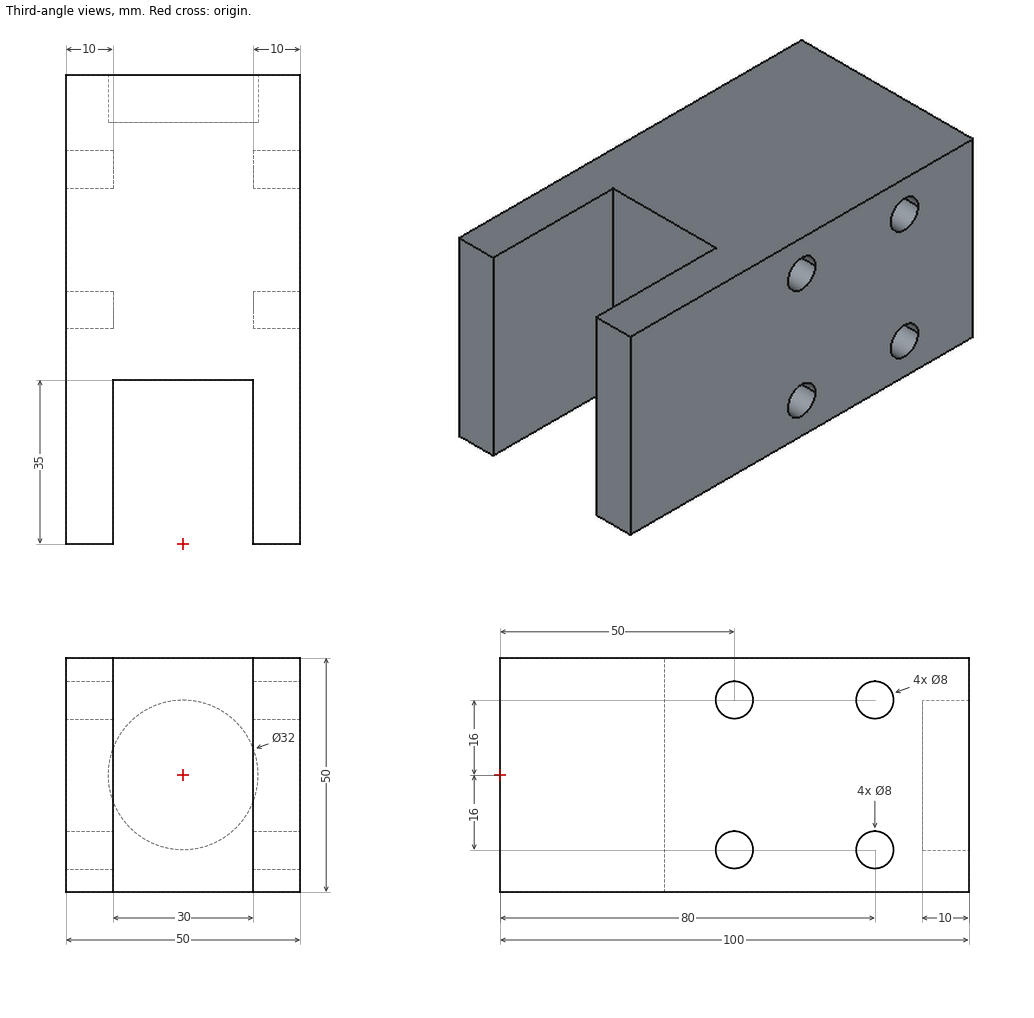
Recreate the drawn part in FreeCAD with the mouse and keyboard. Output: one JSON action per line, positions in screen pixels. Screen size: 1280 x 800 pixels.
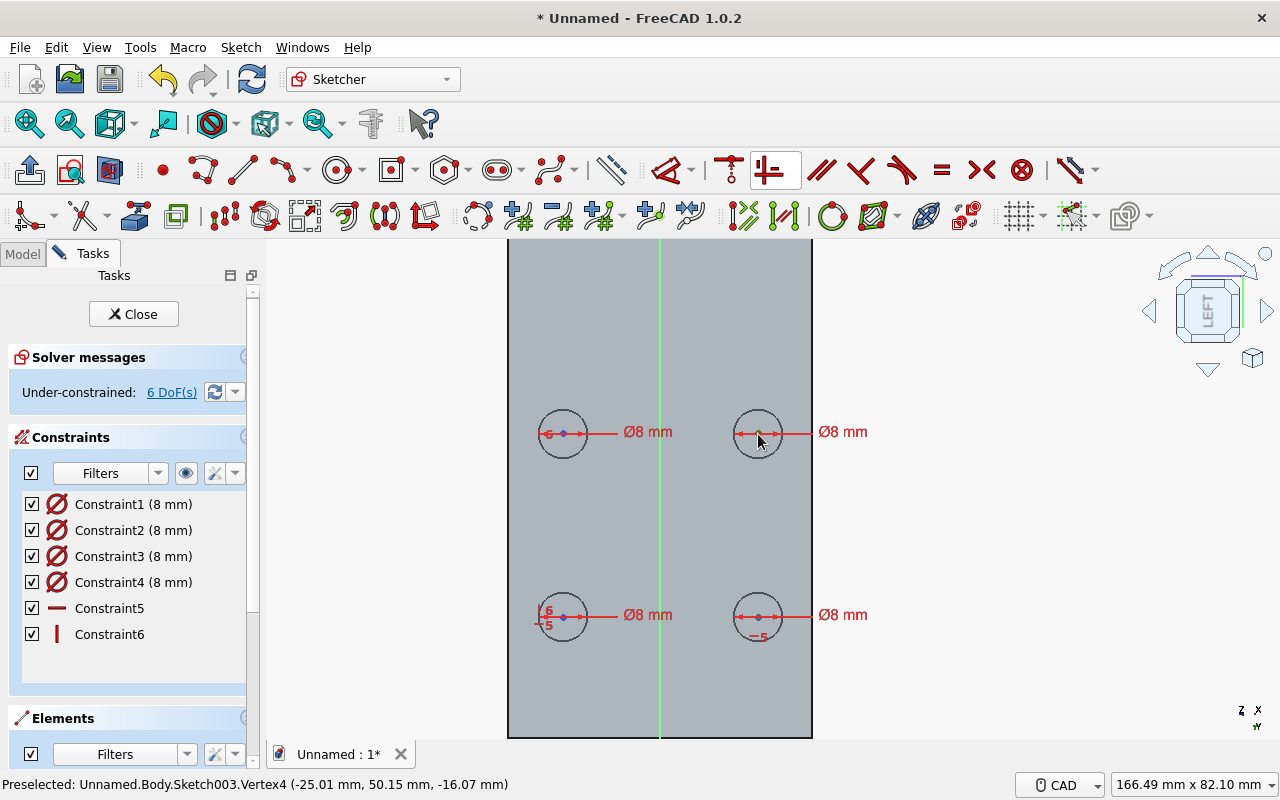
{"action": "left_click", "coordinate": [796, 170]}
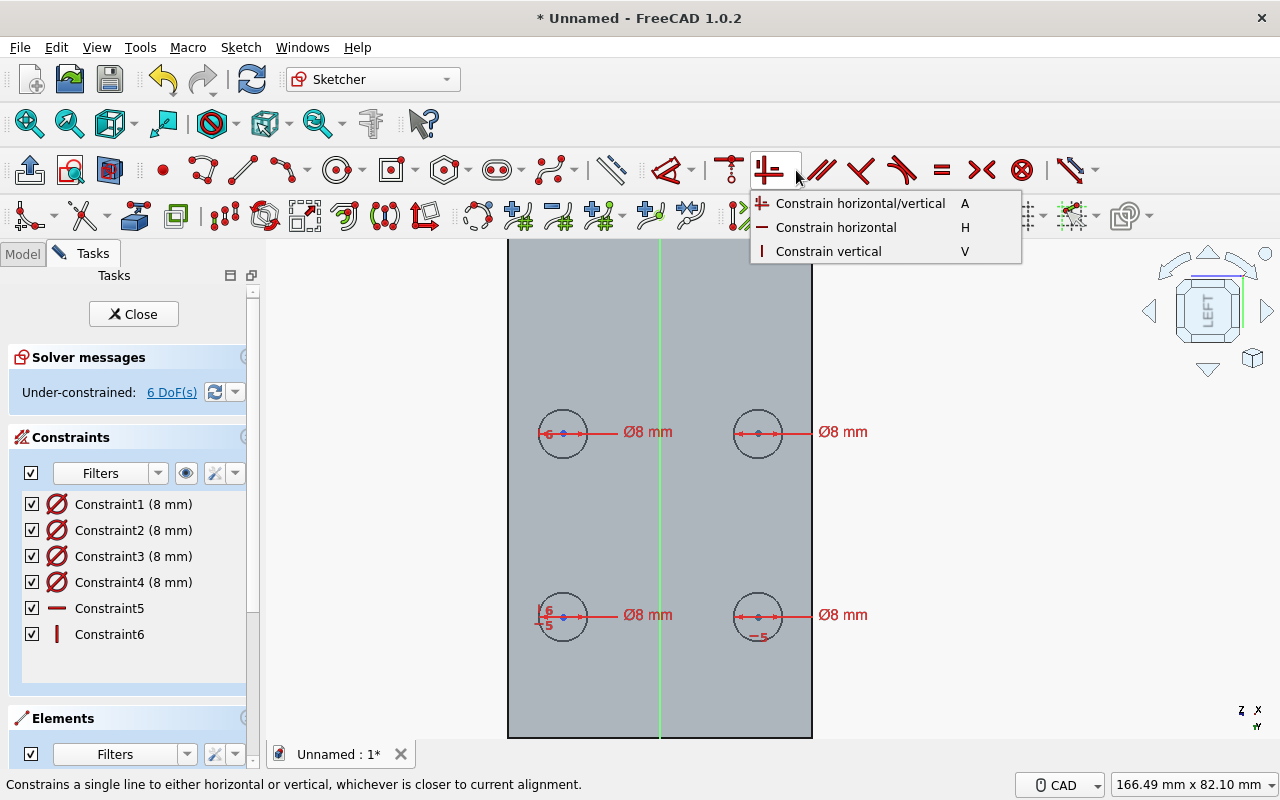
{"action": "left_click", "coordinate": [886, 251]}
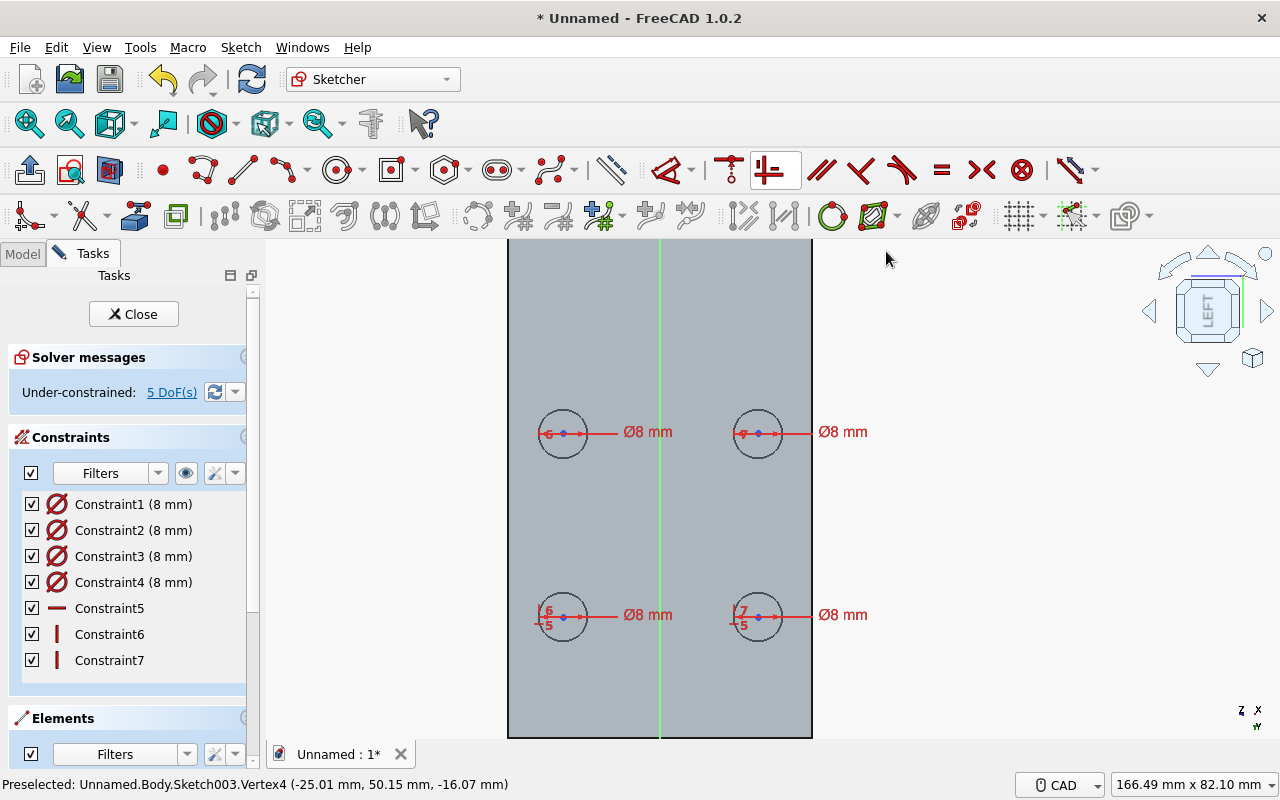
{"action": "left_click", "coordinate": [563, 434]}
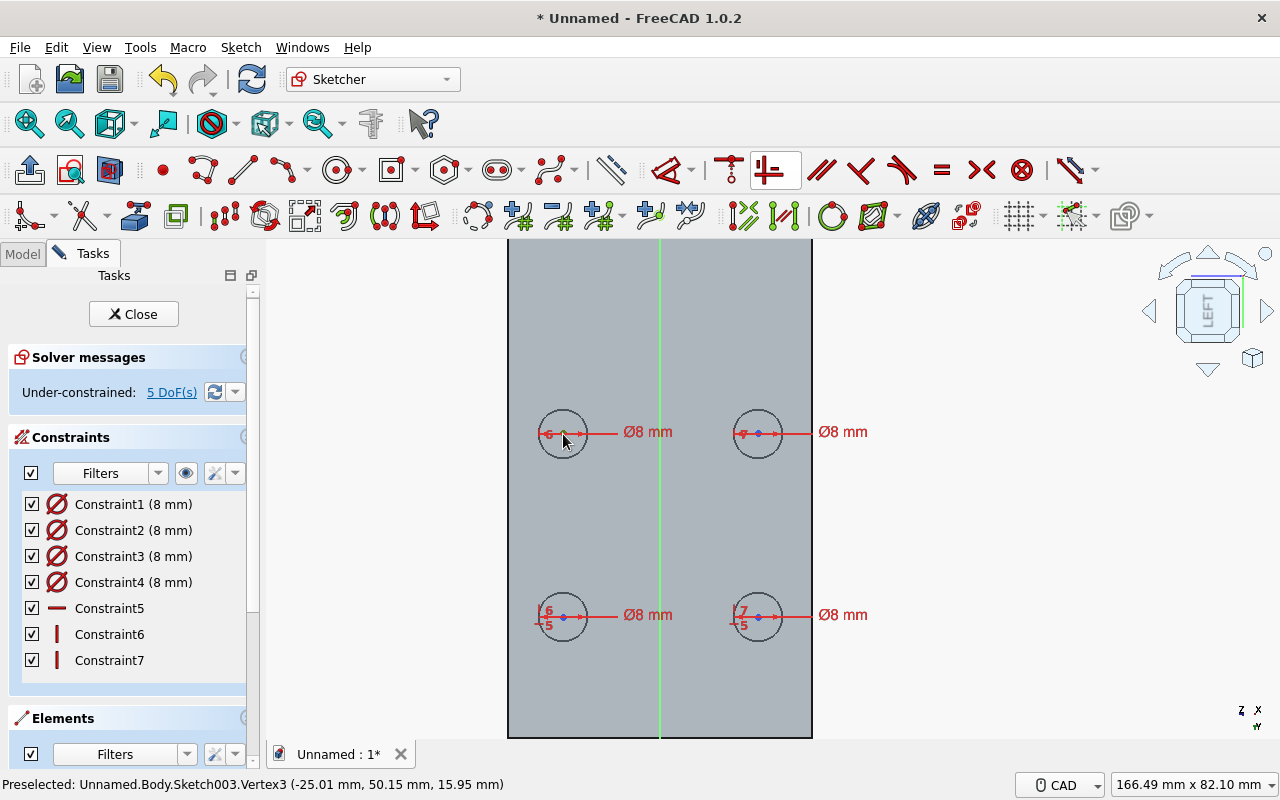
{"action": "left_click", "coordinate": [758, 434]}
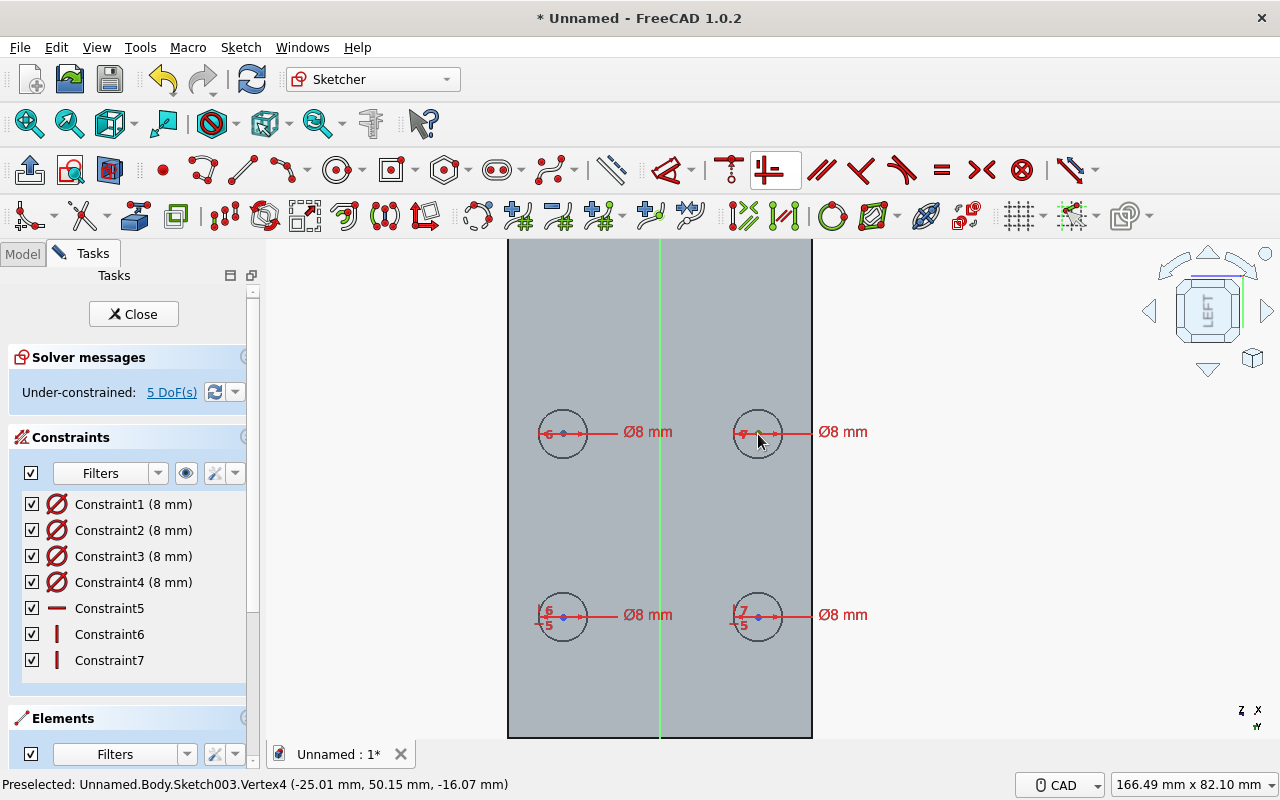
{"action": "key", "text": "h"}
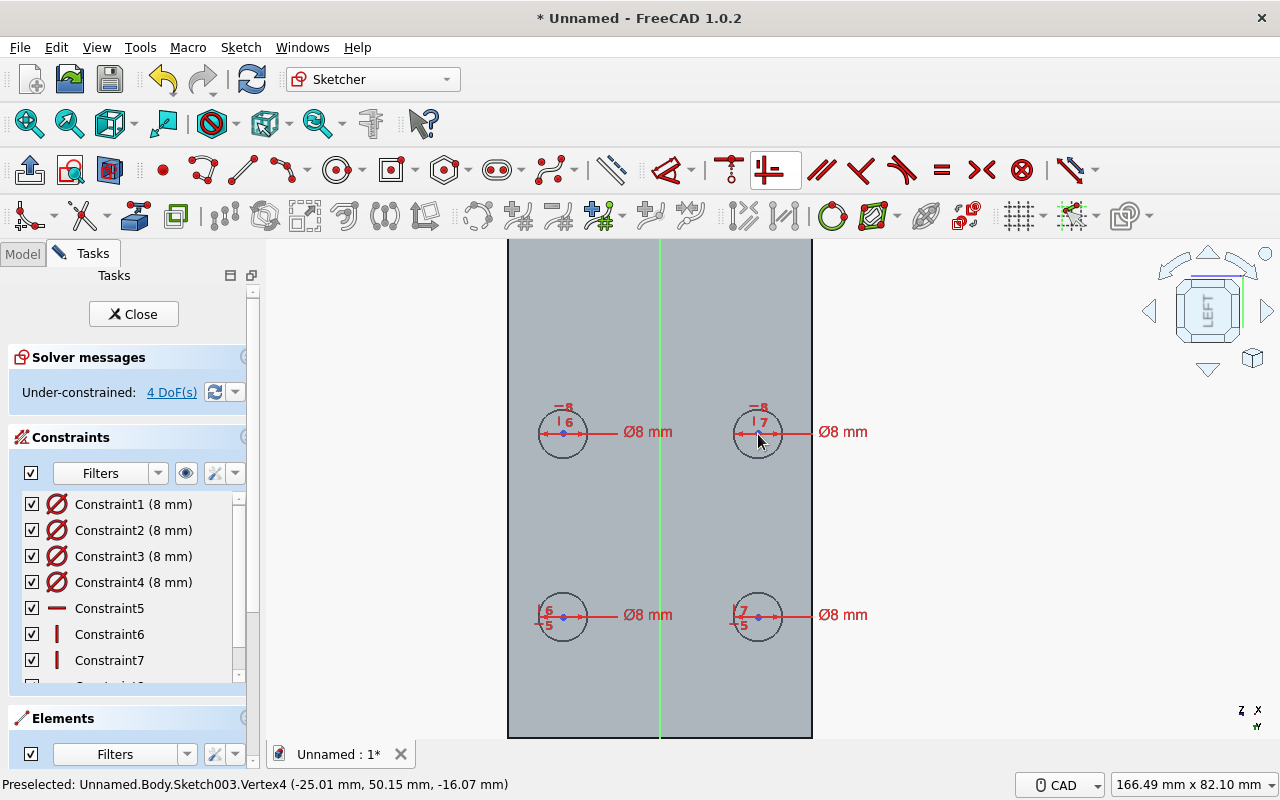
{"action": "left_click", "coordinate": [666, 170]}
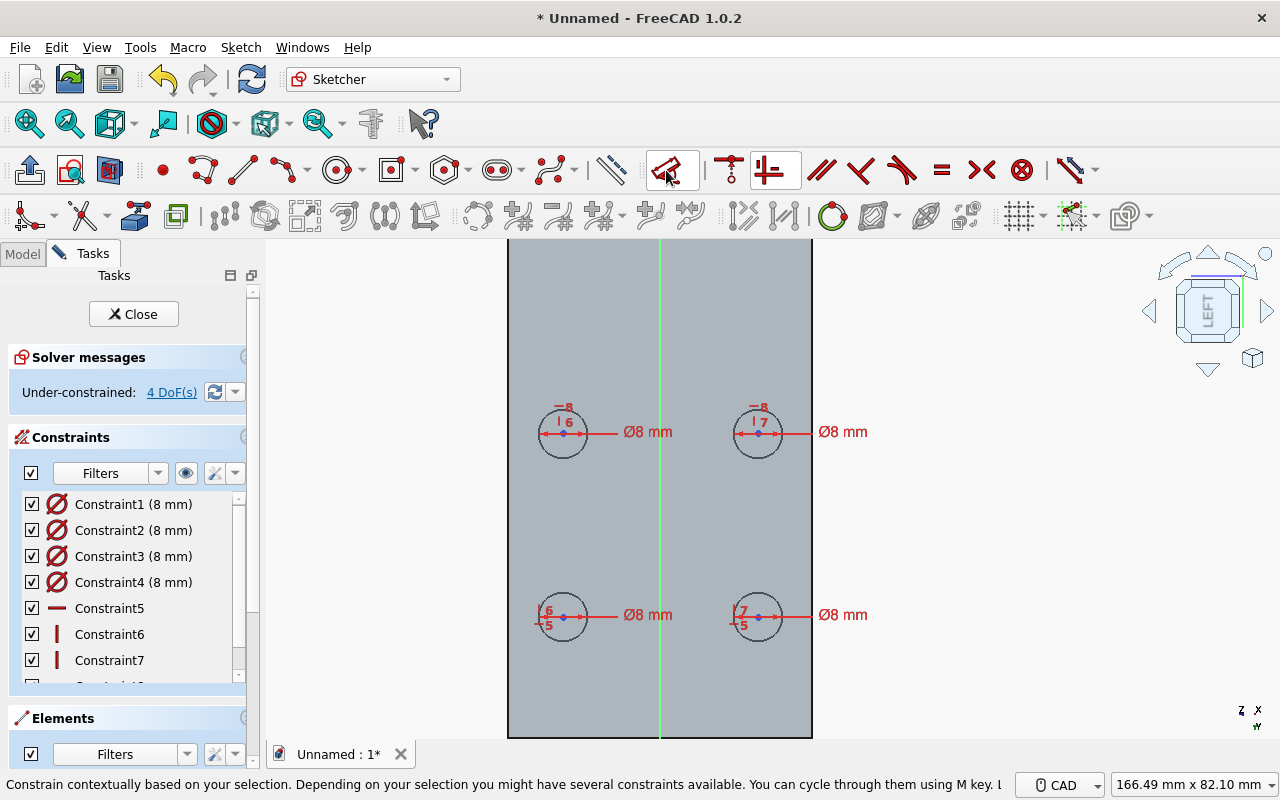
{"action": "left_click", "coordinate": [758, 617]}
{"action": "left_click", "coordinate": [709, 651]}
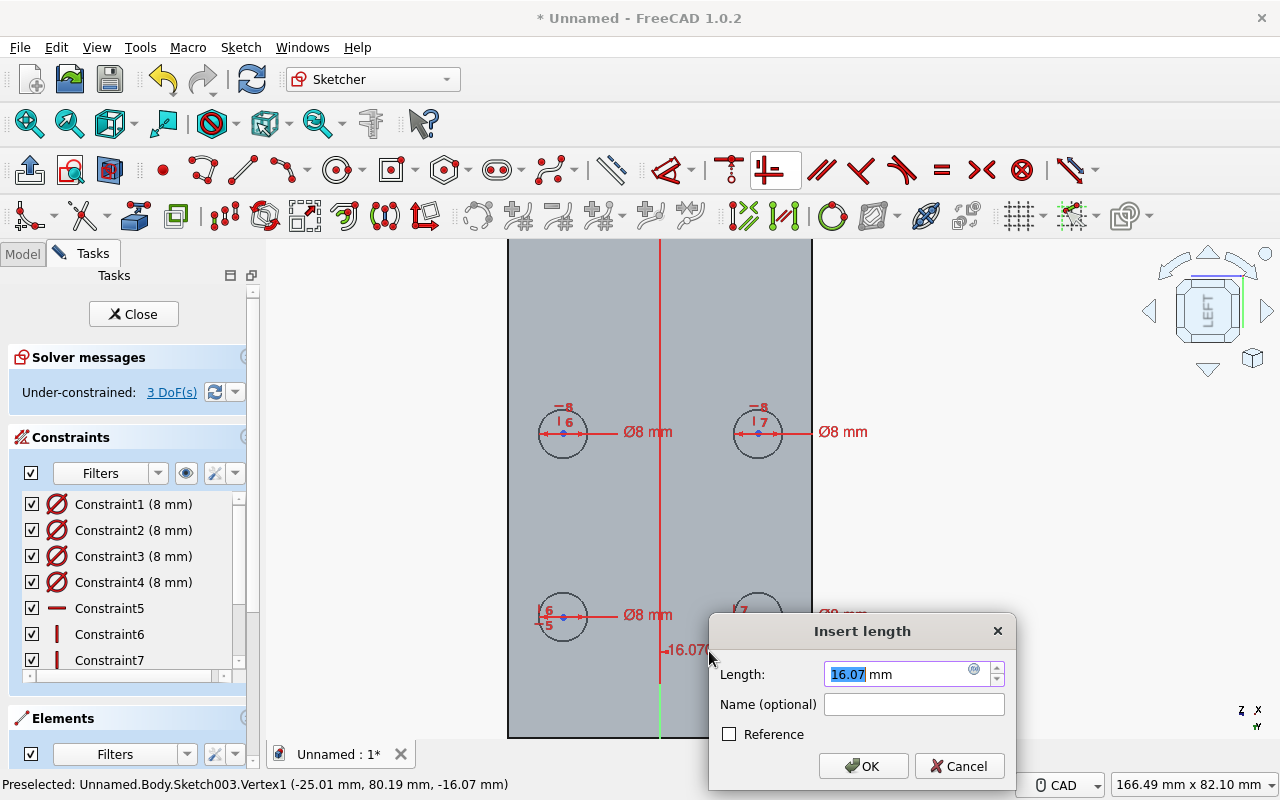
{"action": "type", "text": "16"}
{"action": "key", "text": "Return"}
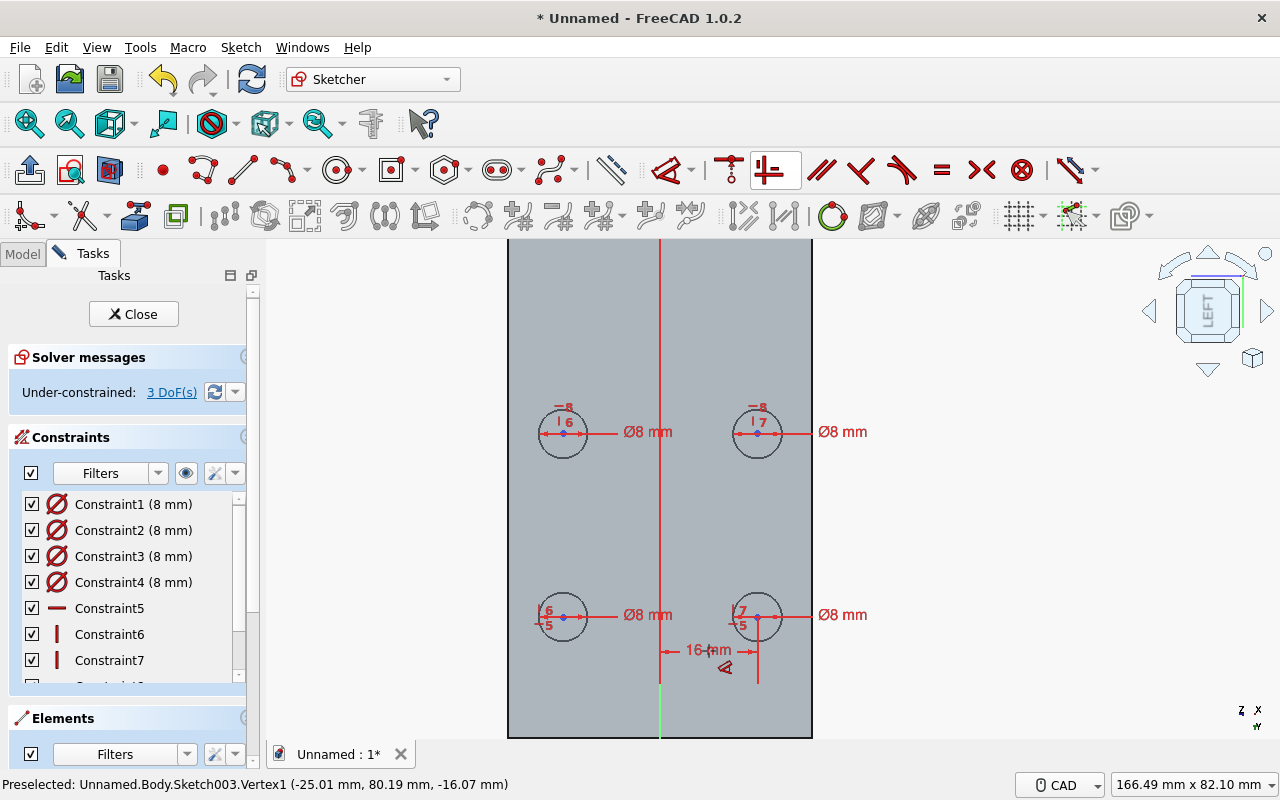
{"action": "left_click", "coordinate": [758, 617]}
{"action": "left_click", "coordinate": [792, 361]}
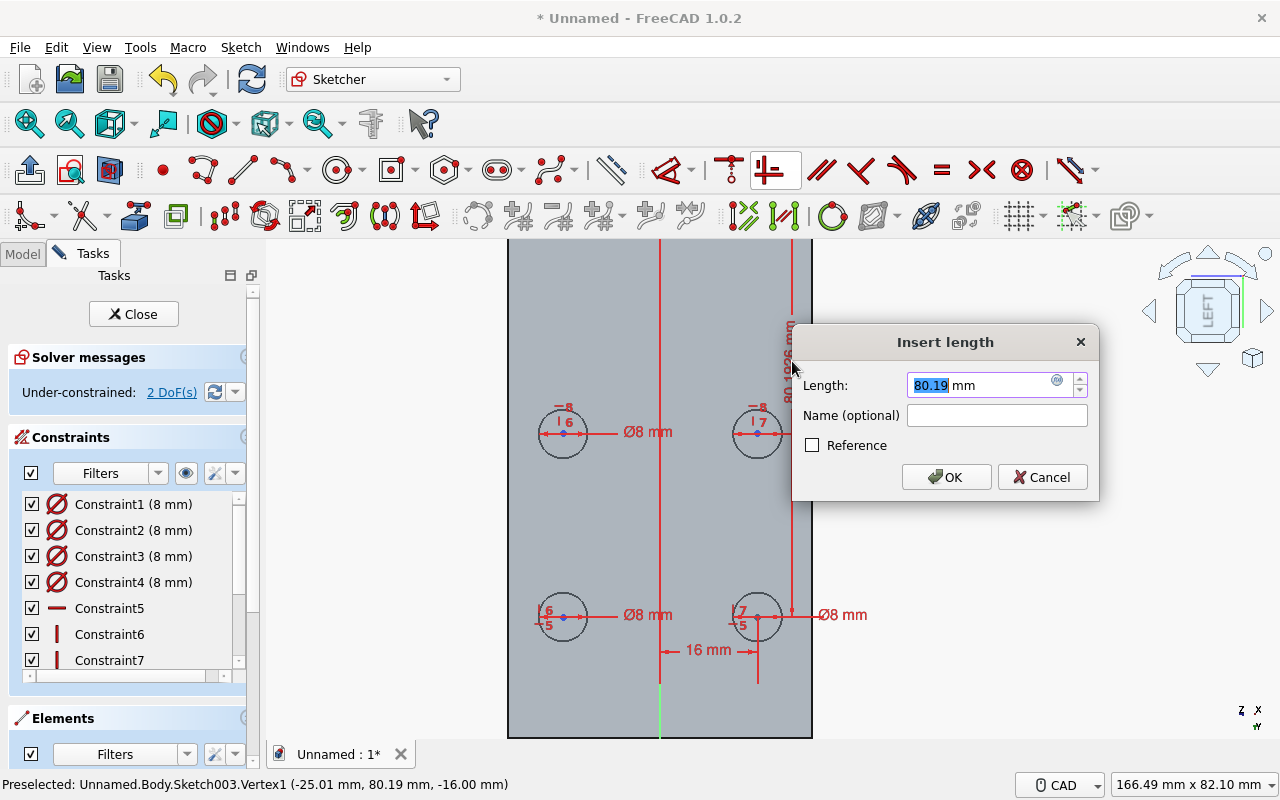
{"action": "type", "text": "80"}
{"action": "key", "text": "Return"}